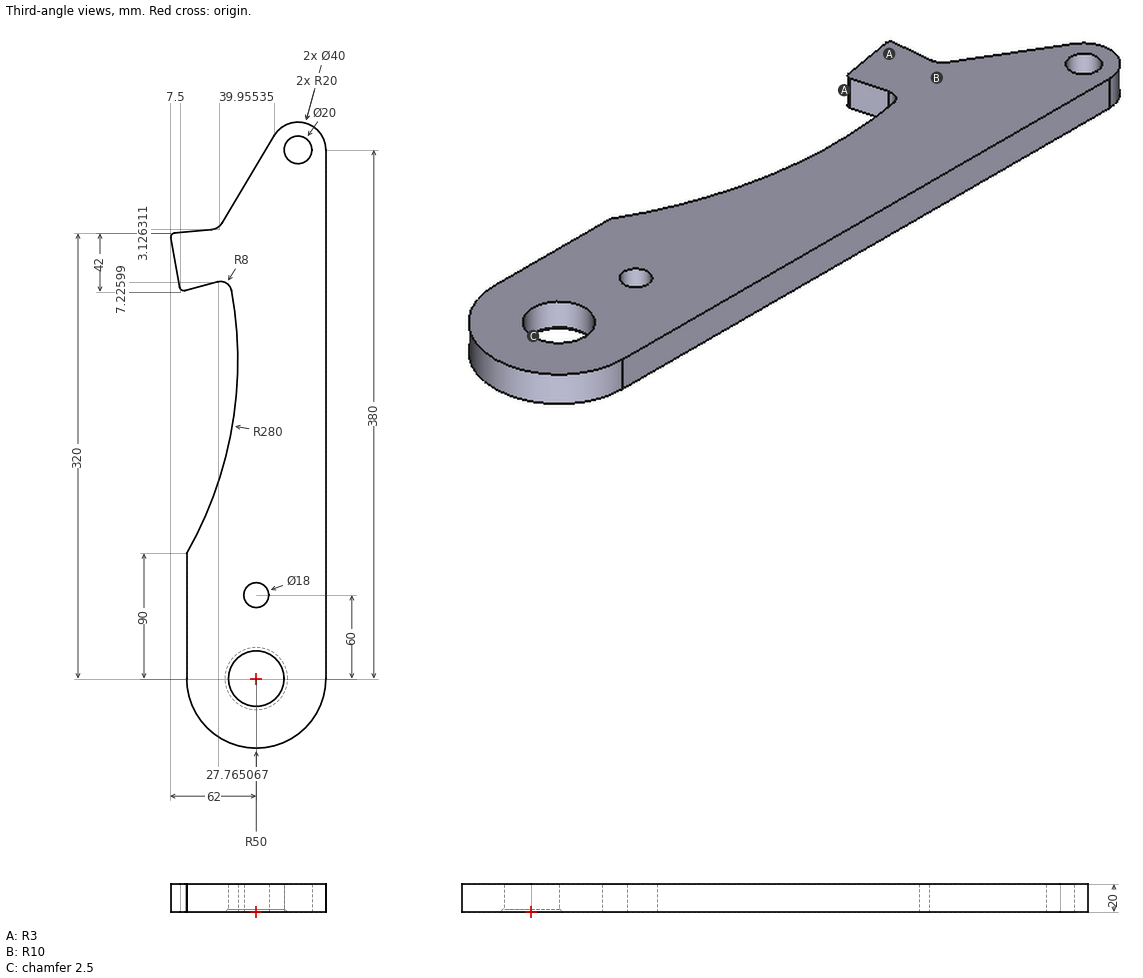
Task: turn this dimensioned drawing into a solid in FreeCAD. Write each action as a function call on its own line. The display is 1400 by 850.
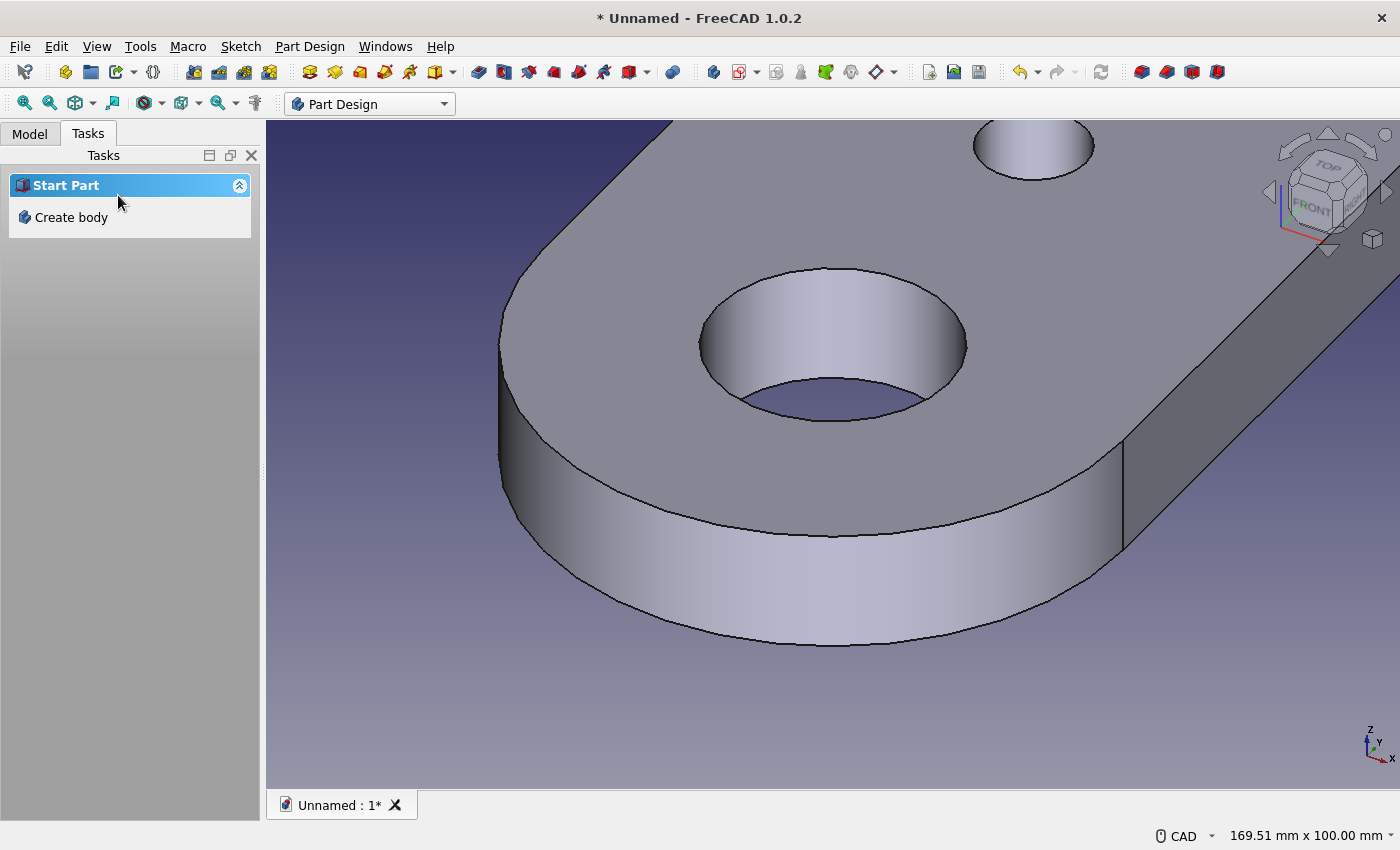
click(25, 104)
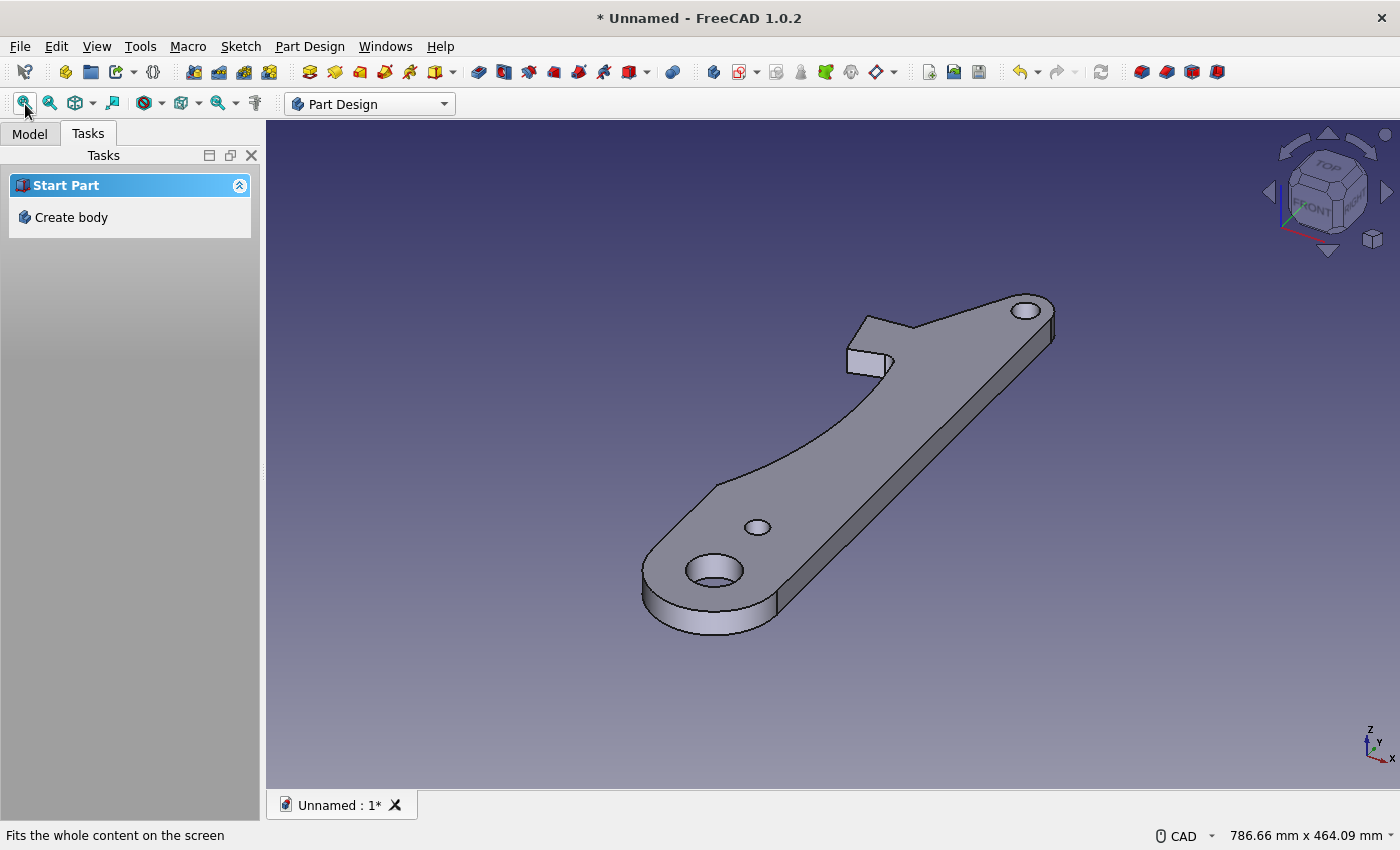
key(0)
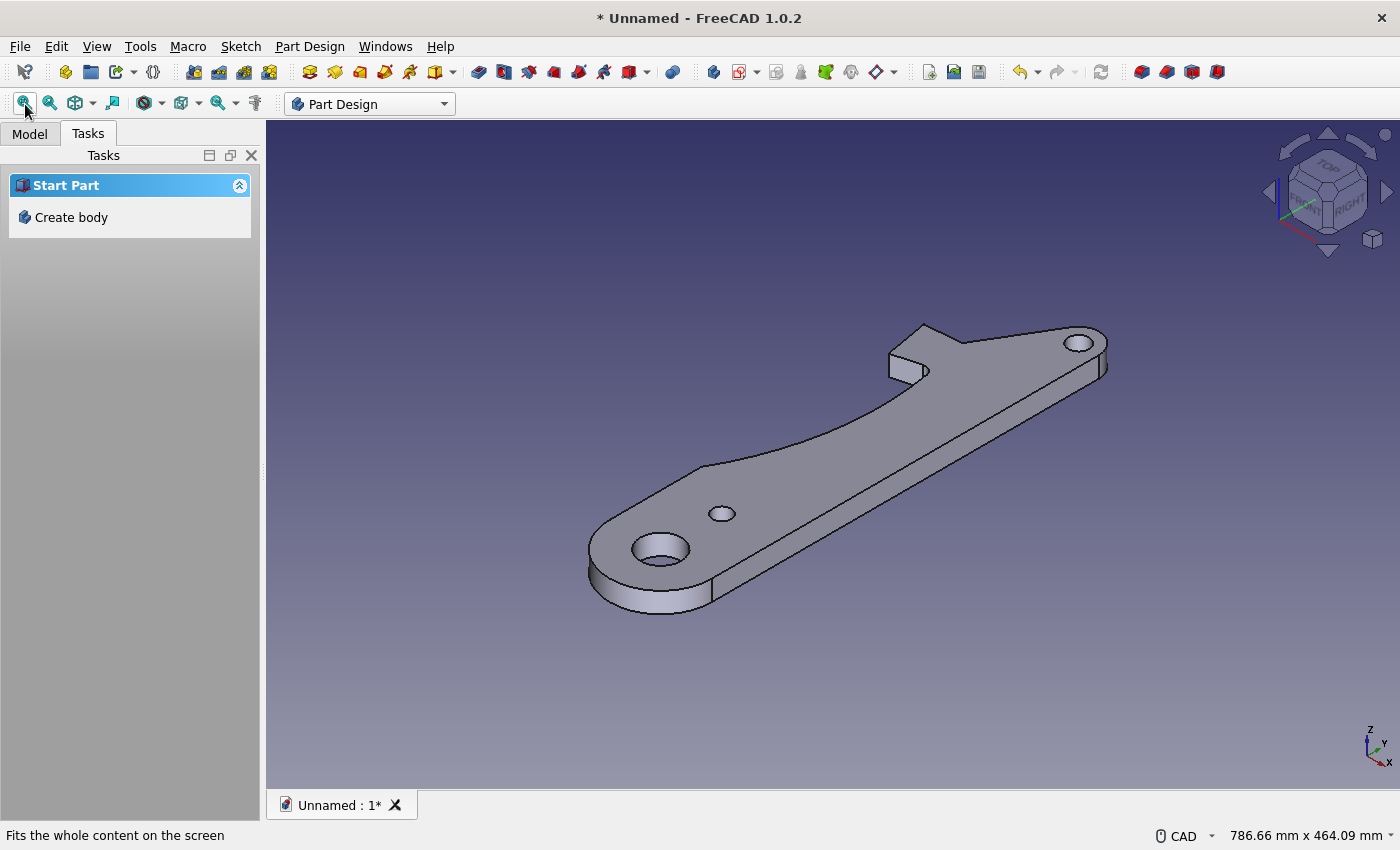
key(2)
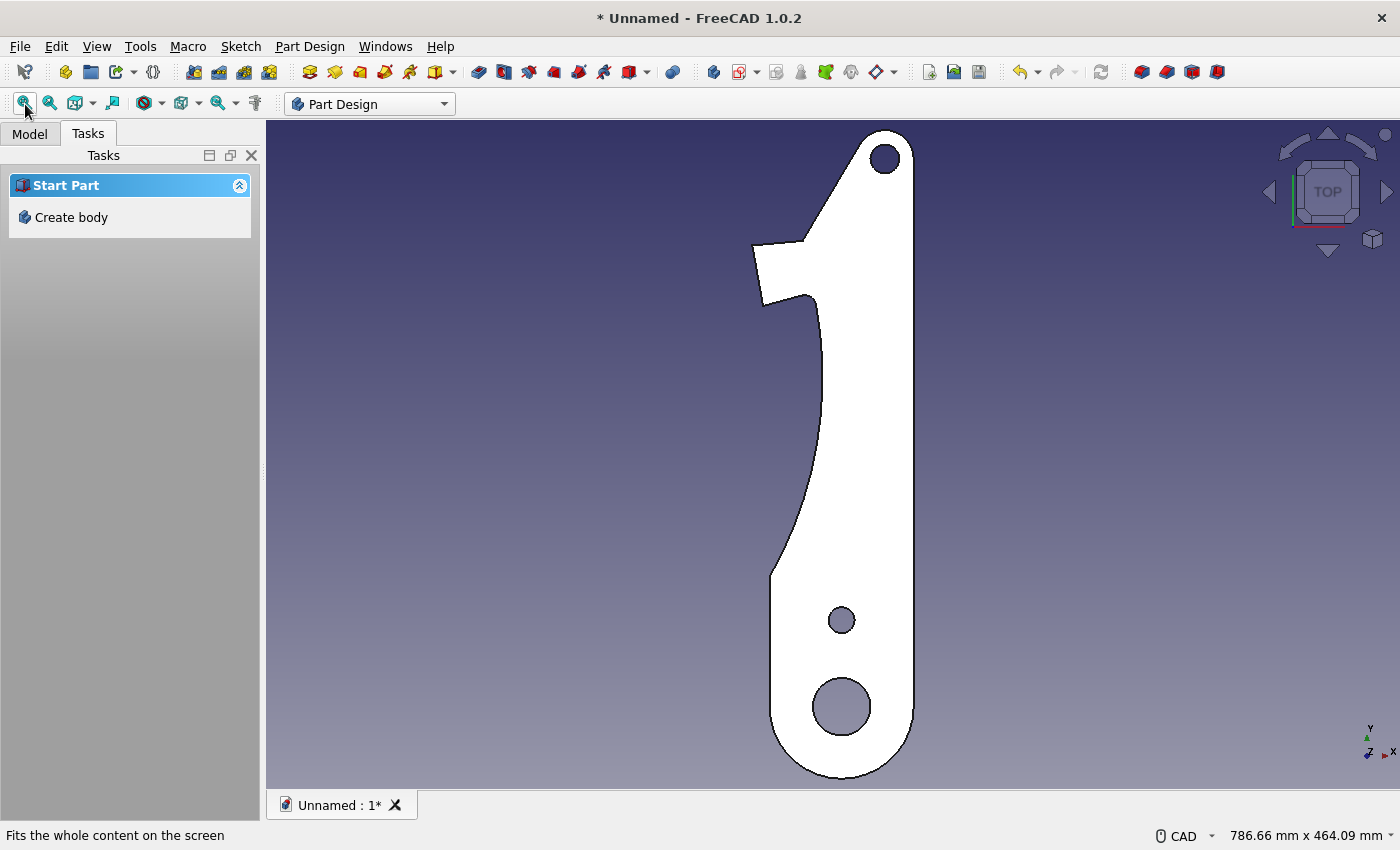
key(1)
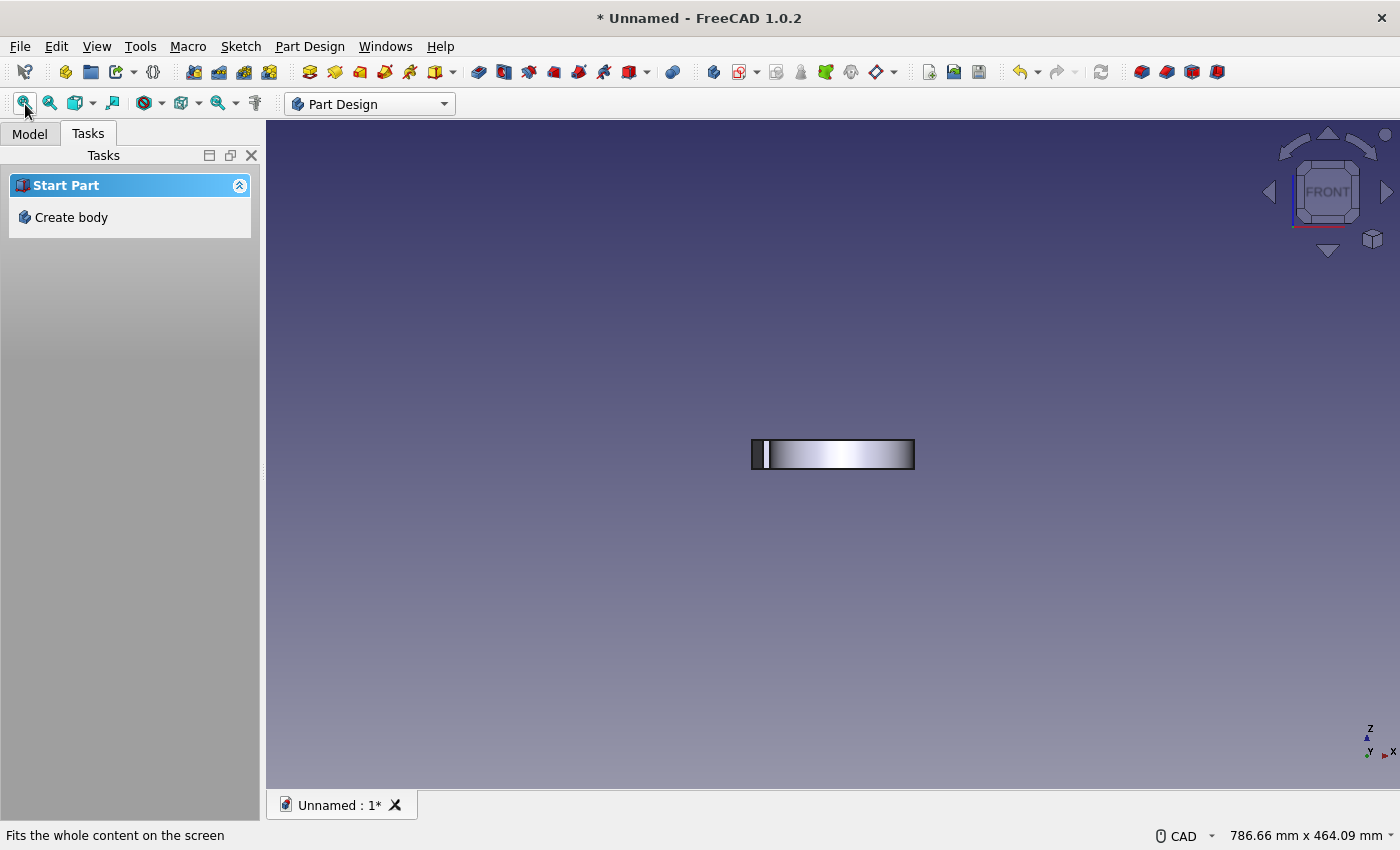
click(25, 104)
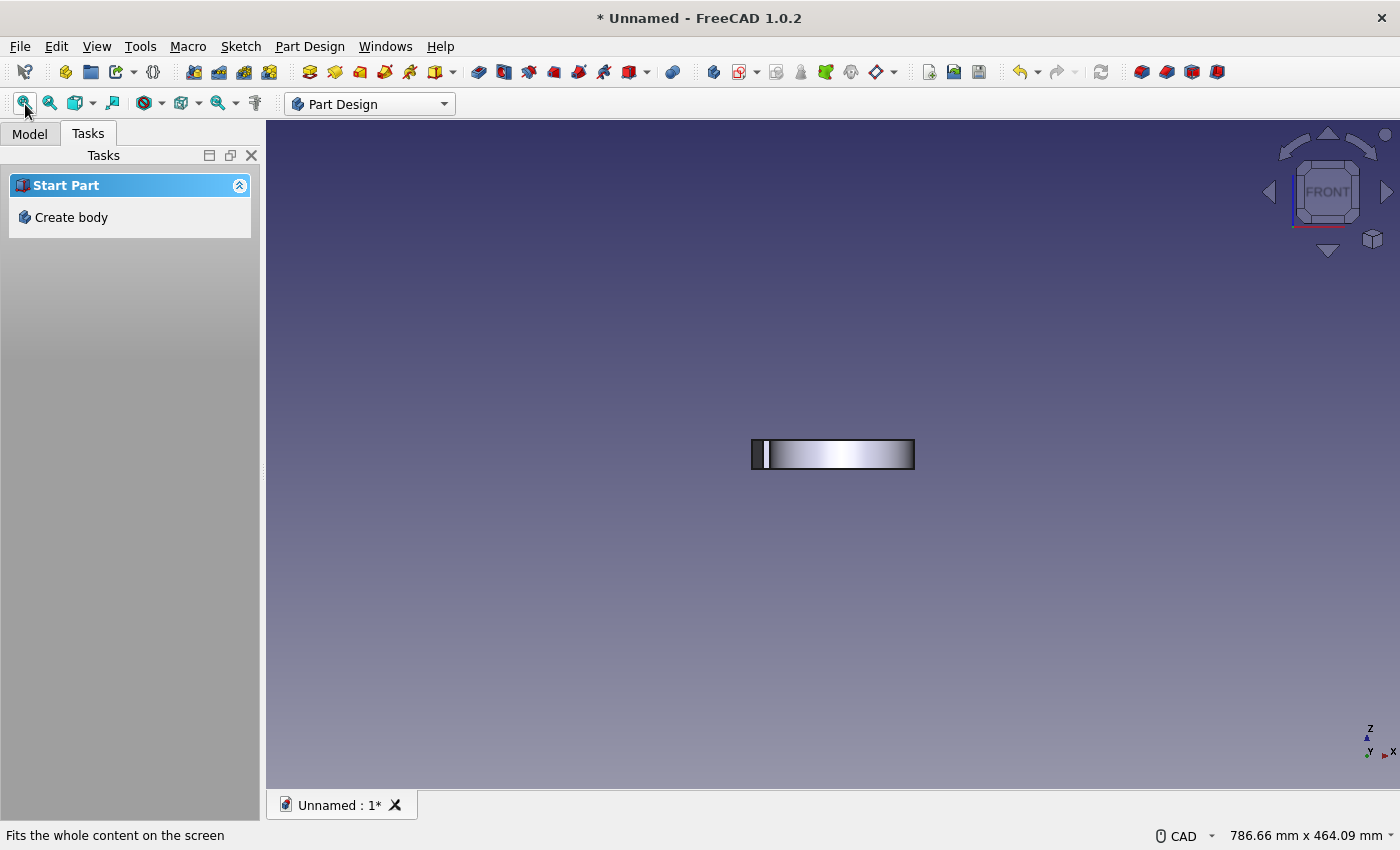
click(763, 454)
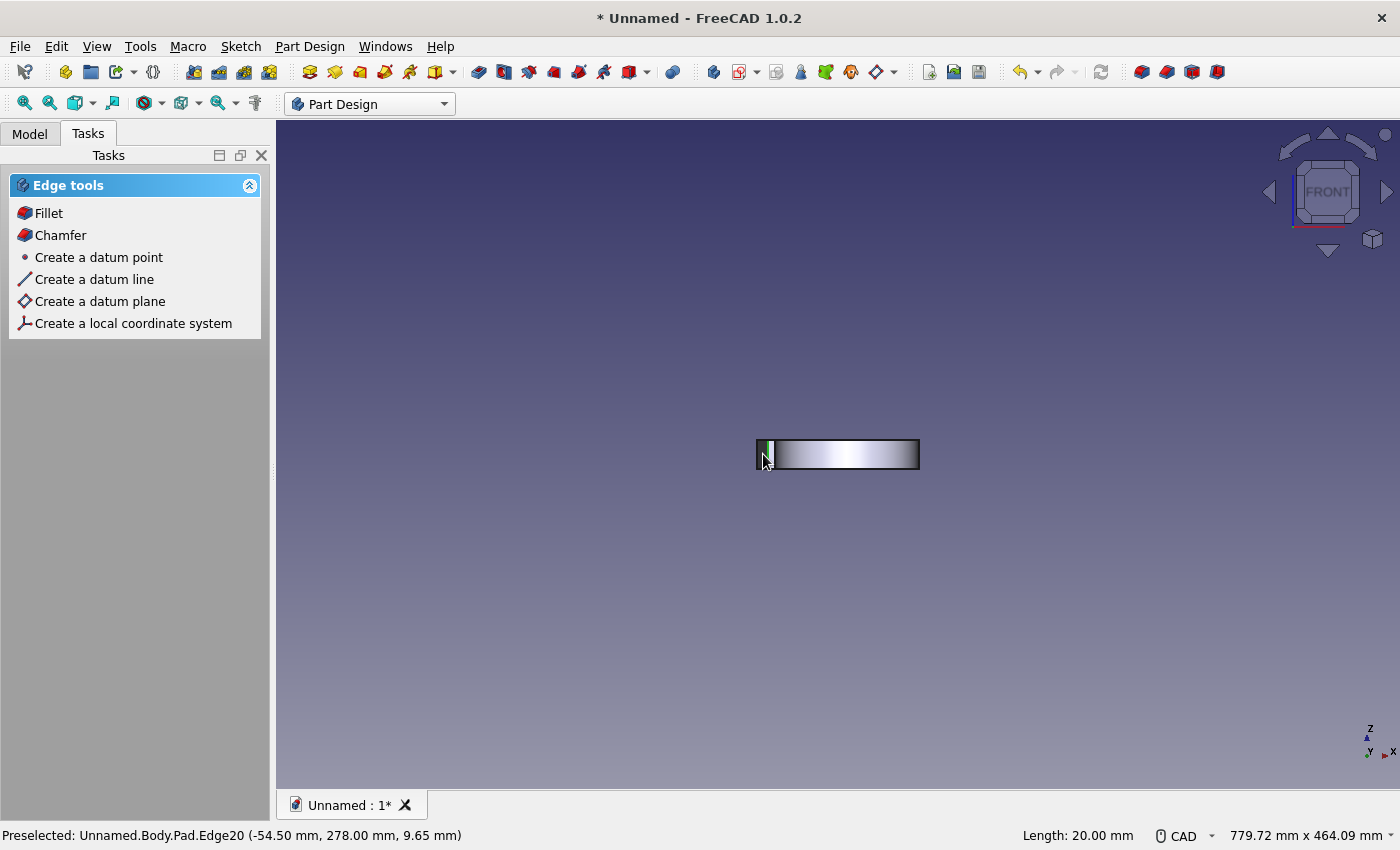
key(3)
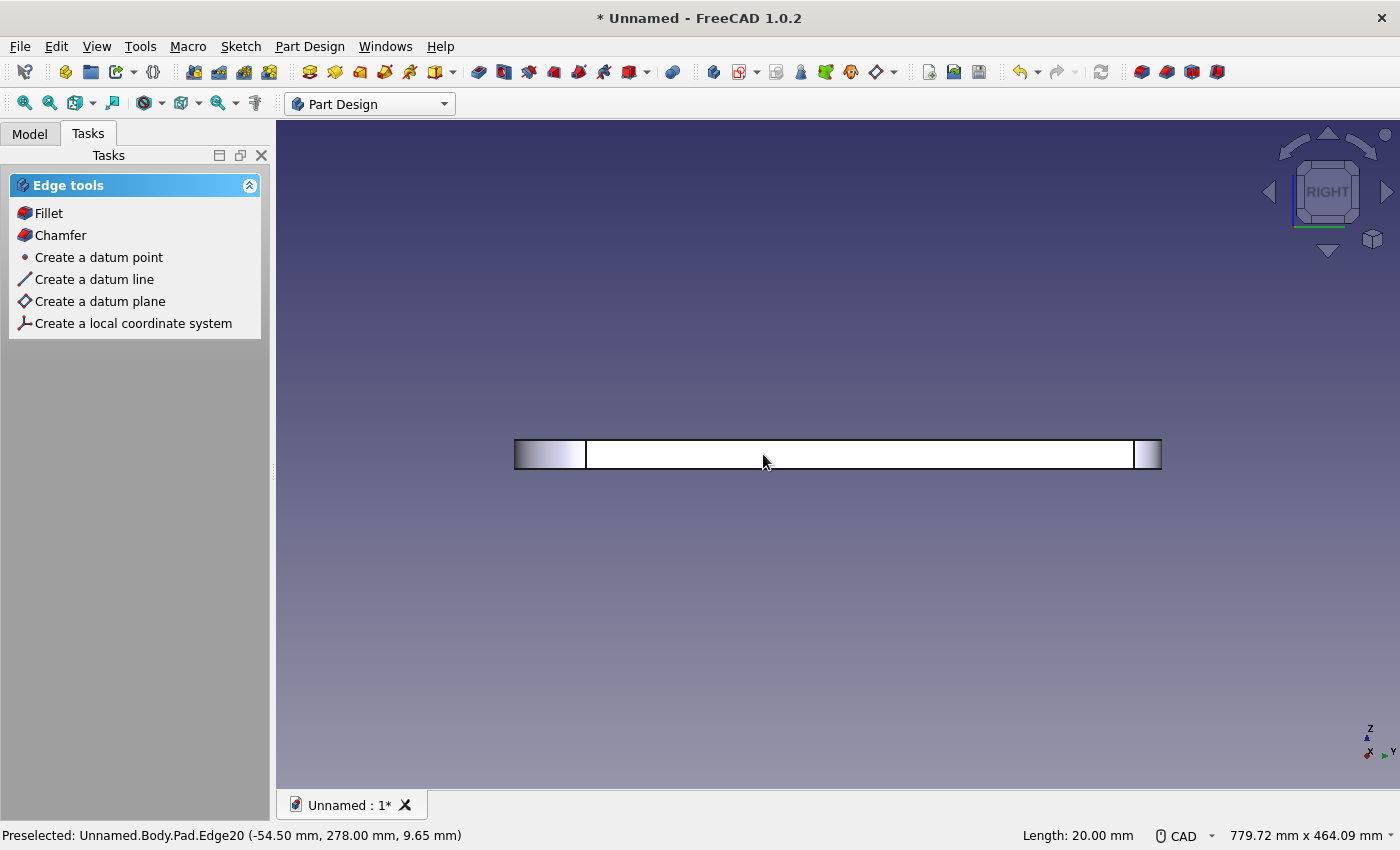
key(5)